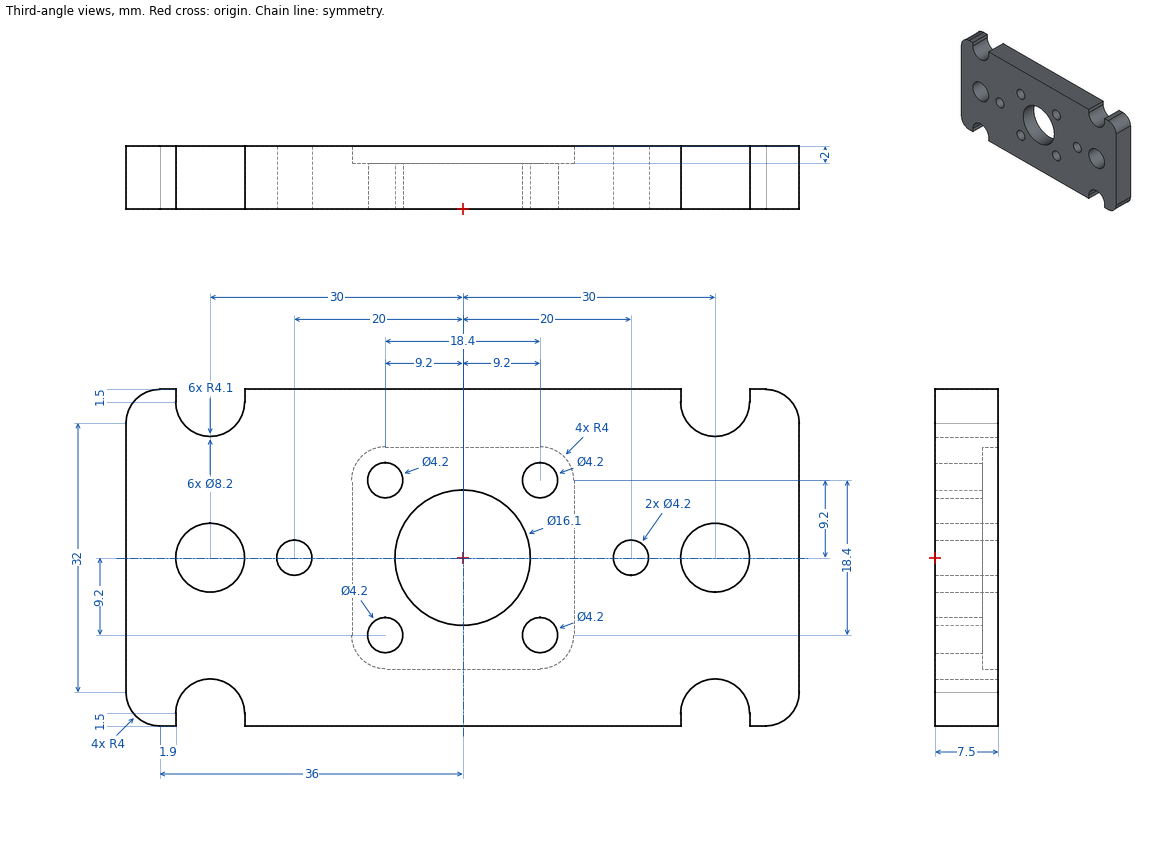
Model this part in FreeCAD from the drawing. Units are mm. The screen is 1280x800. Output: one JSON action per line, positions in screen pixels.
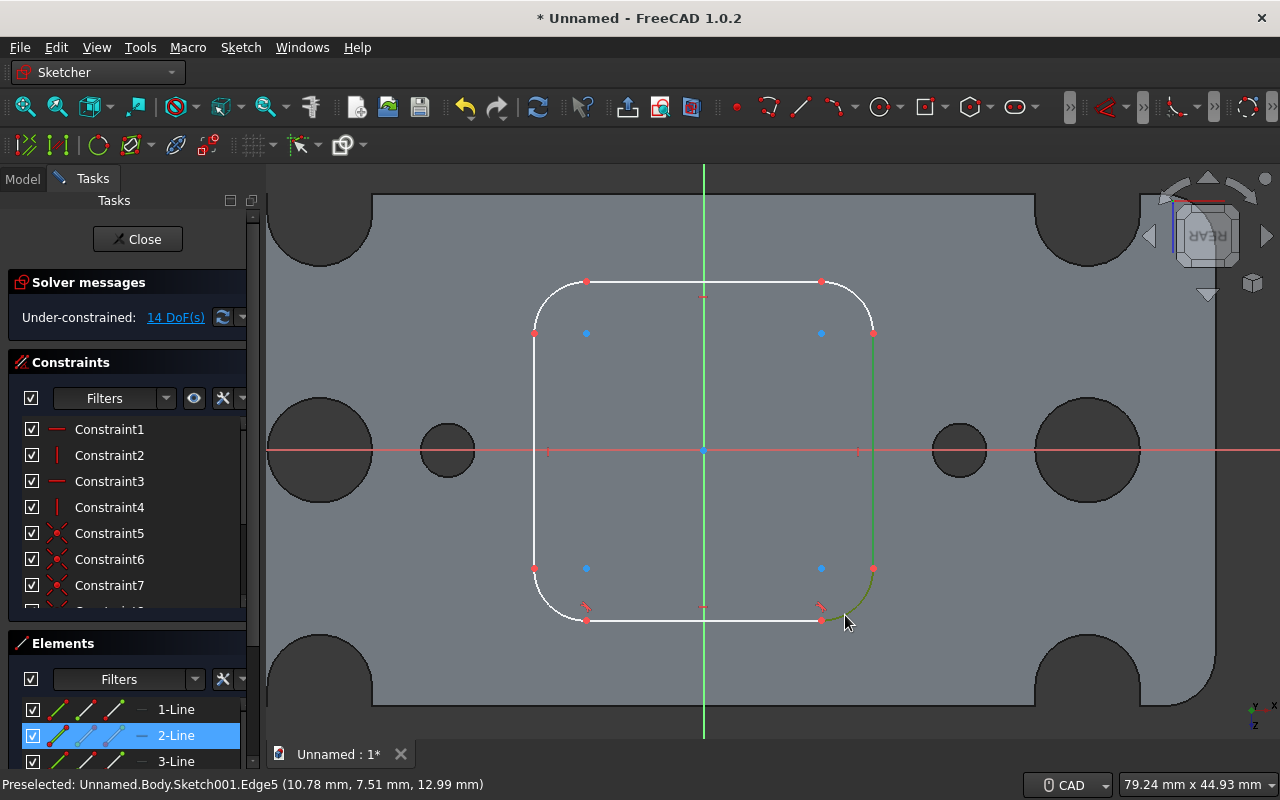
{"action": "key", "text": "t"}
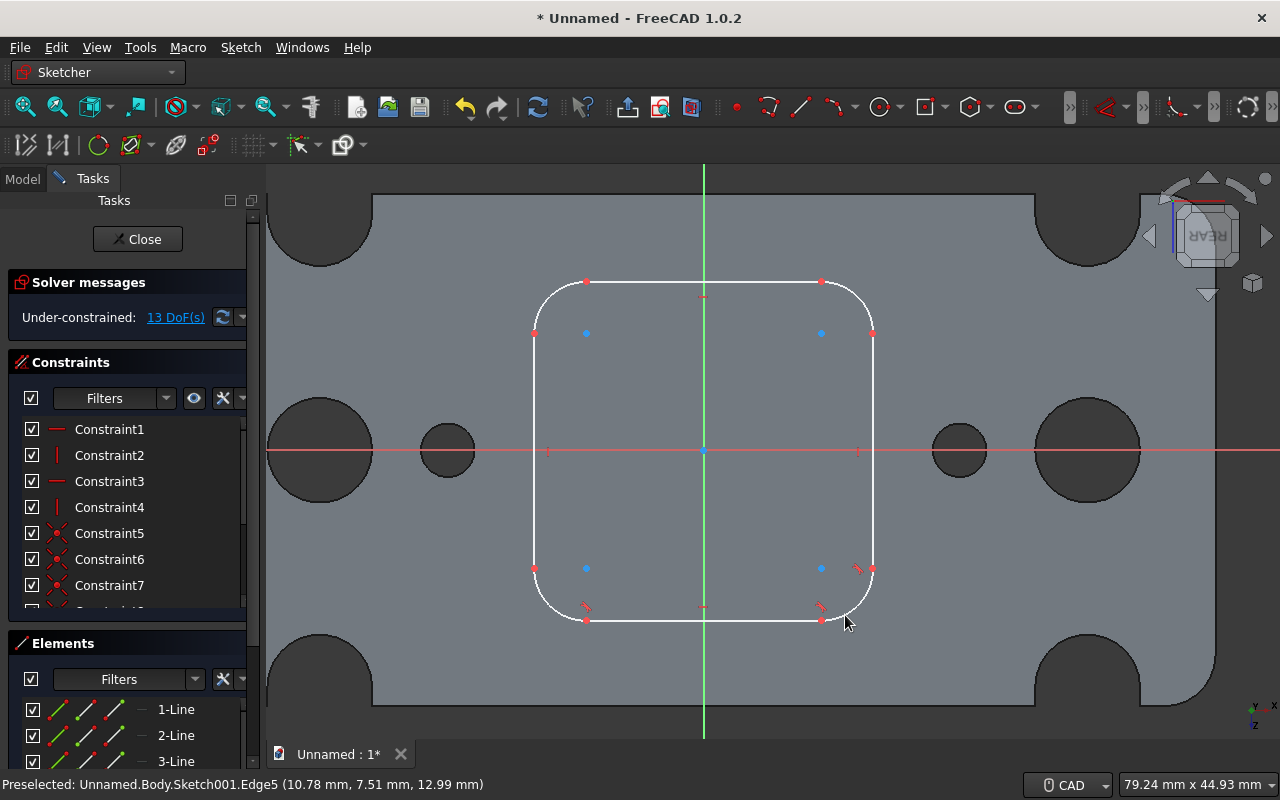
{"action": "left_click", "coordinate": [873, 498]}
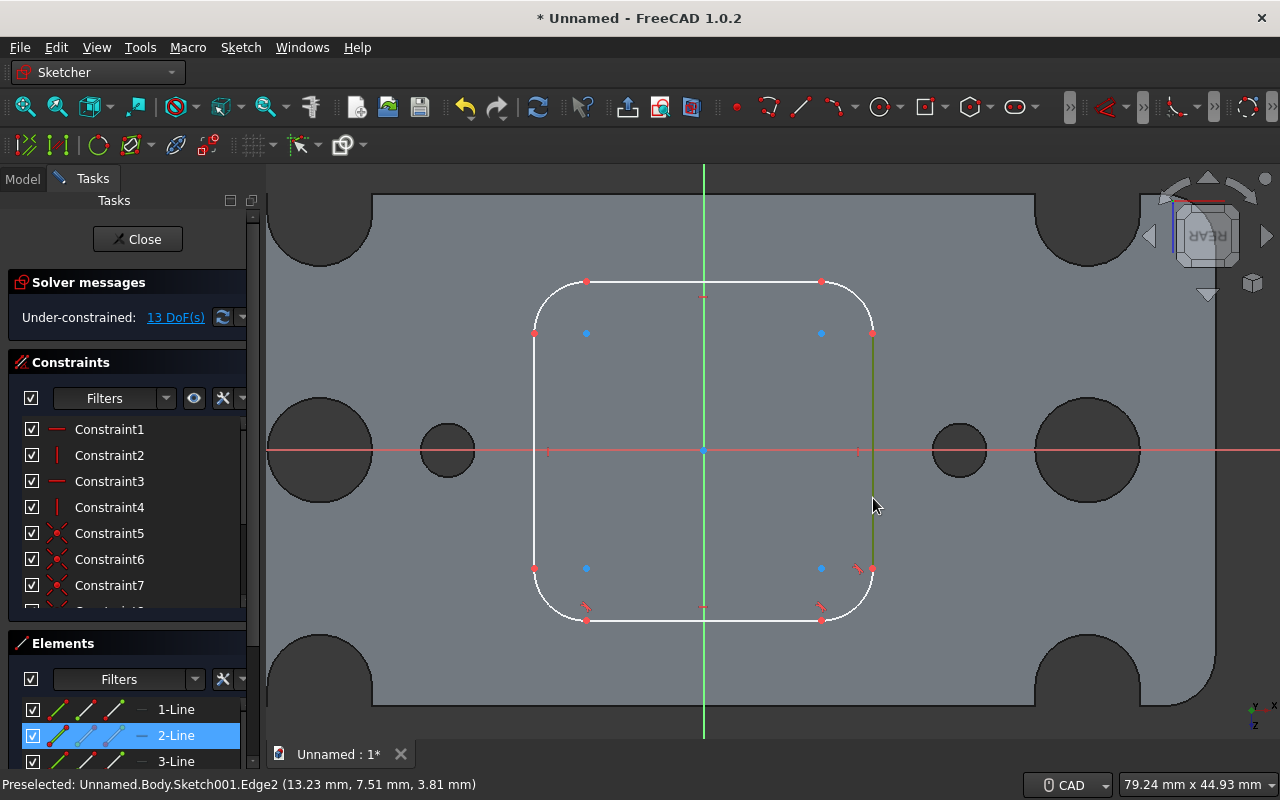
{"action": "left_click", "coordinate": [868, 310]}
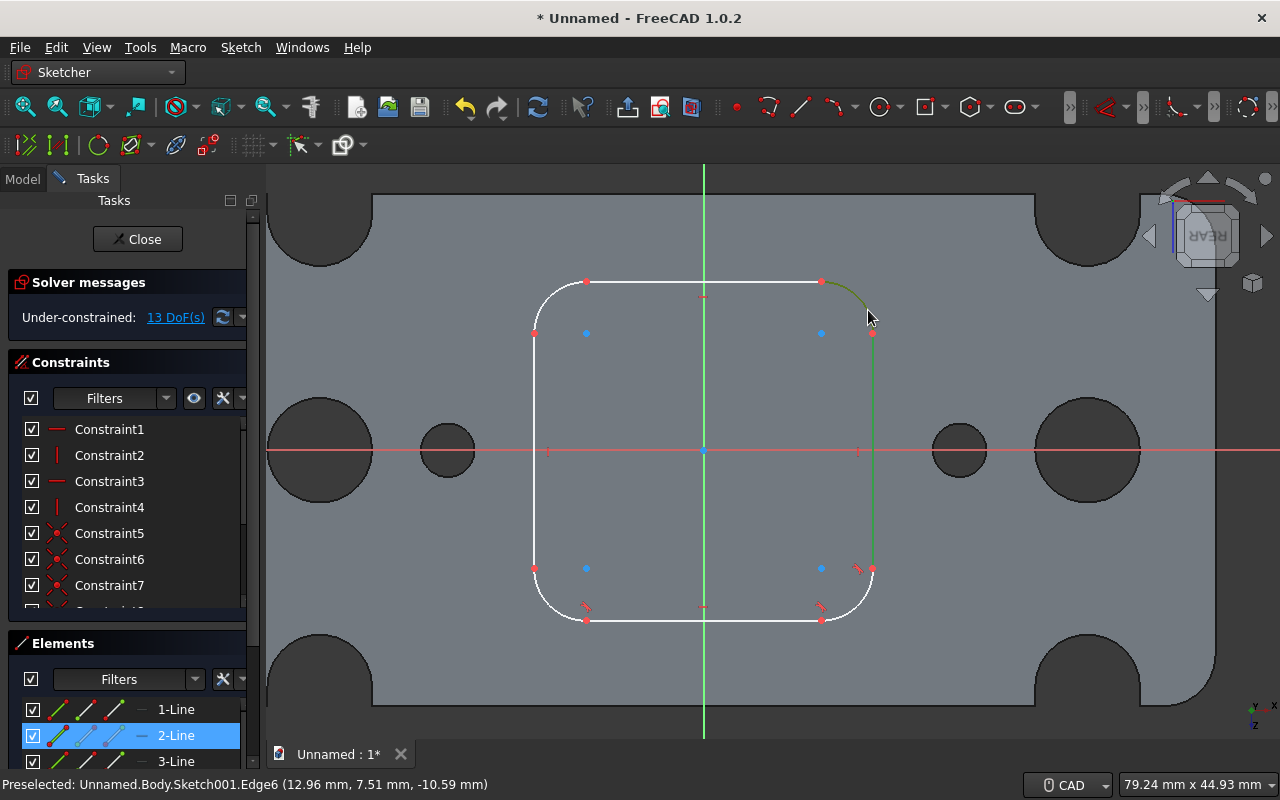
{"action": "key", "text": "t"}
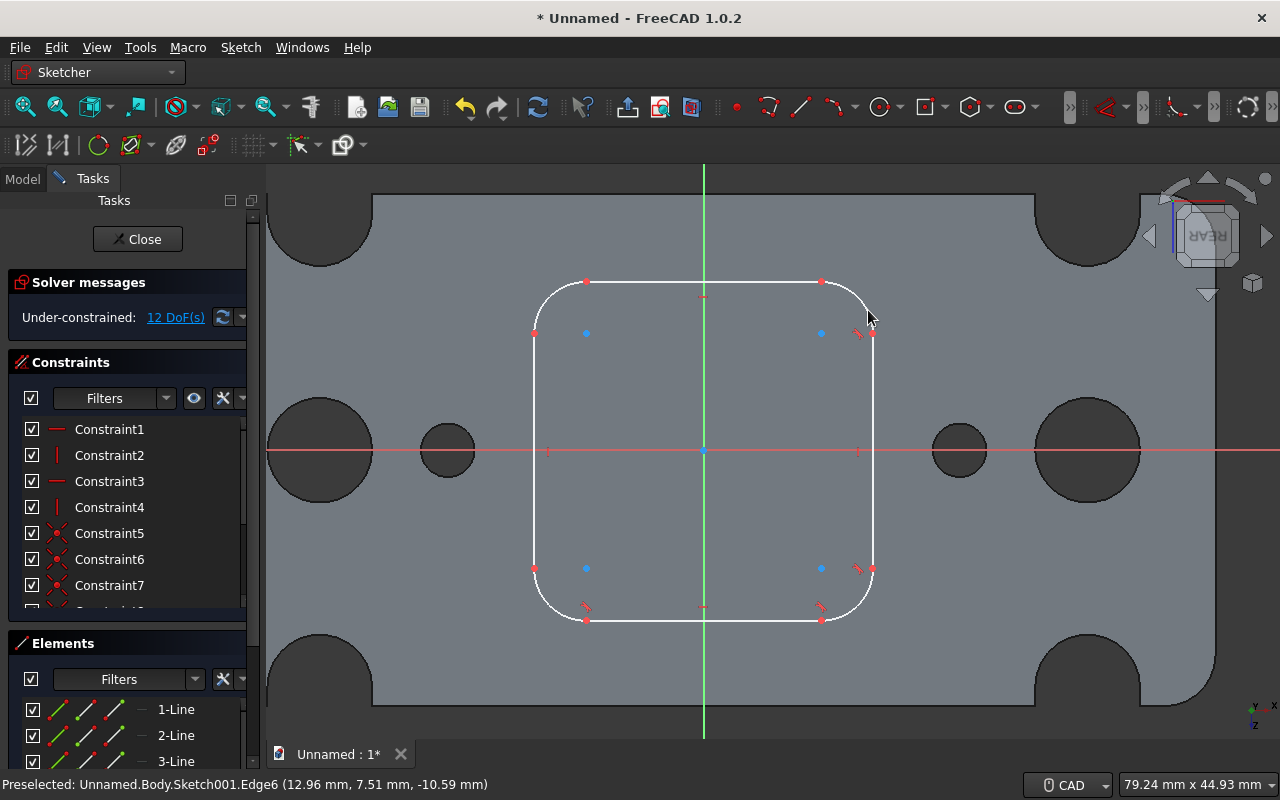
{"action": "left_click", "coordinate": [750, 282]}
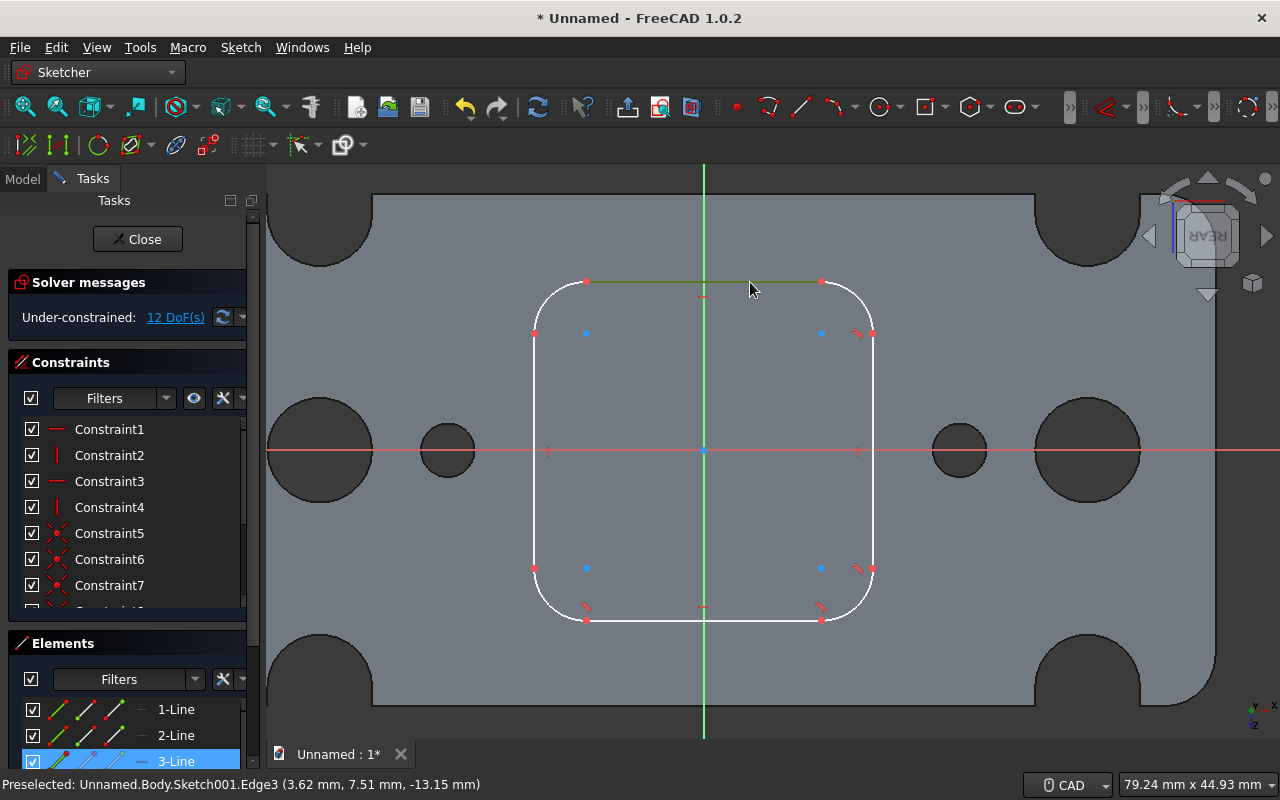
{"action": "left_click", "coordinate": [867, 310]}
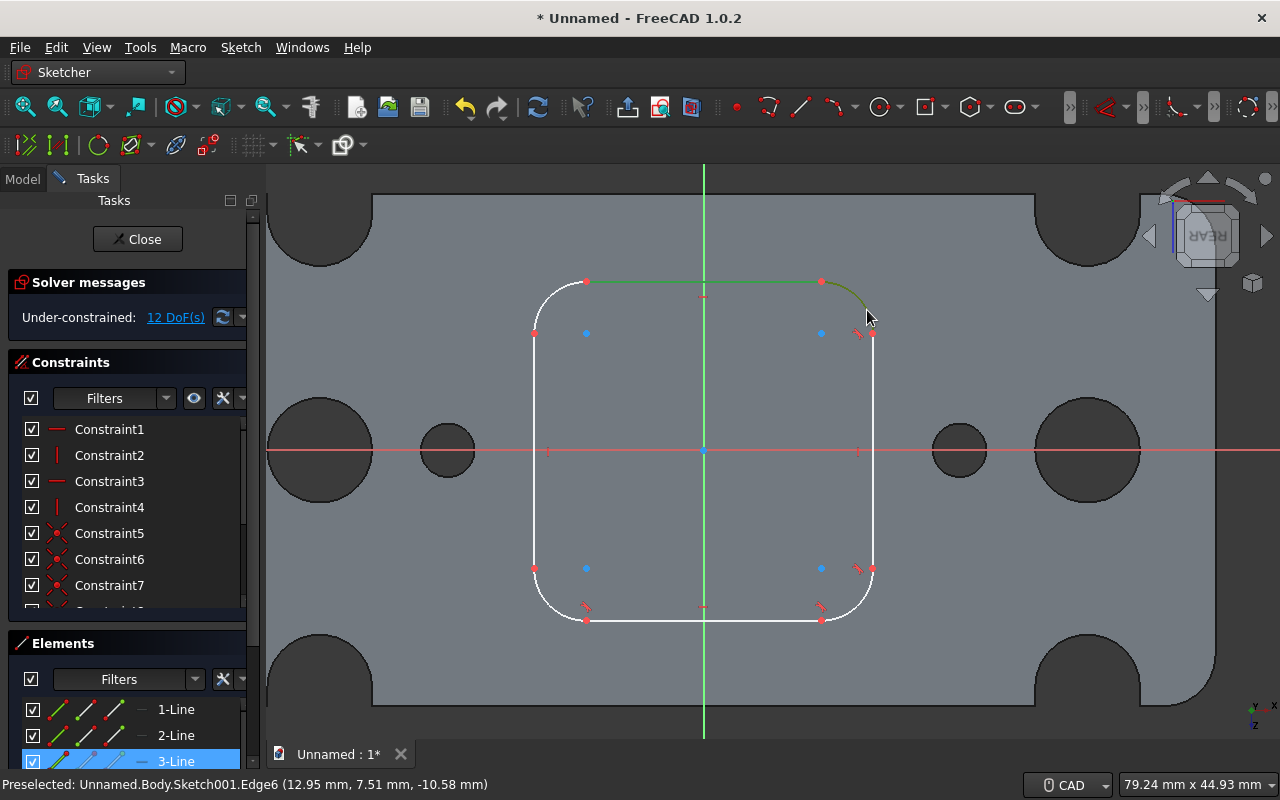
{"action": "key", "text": "t"}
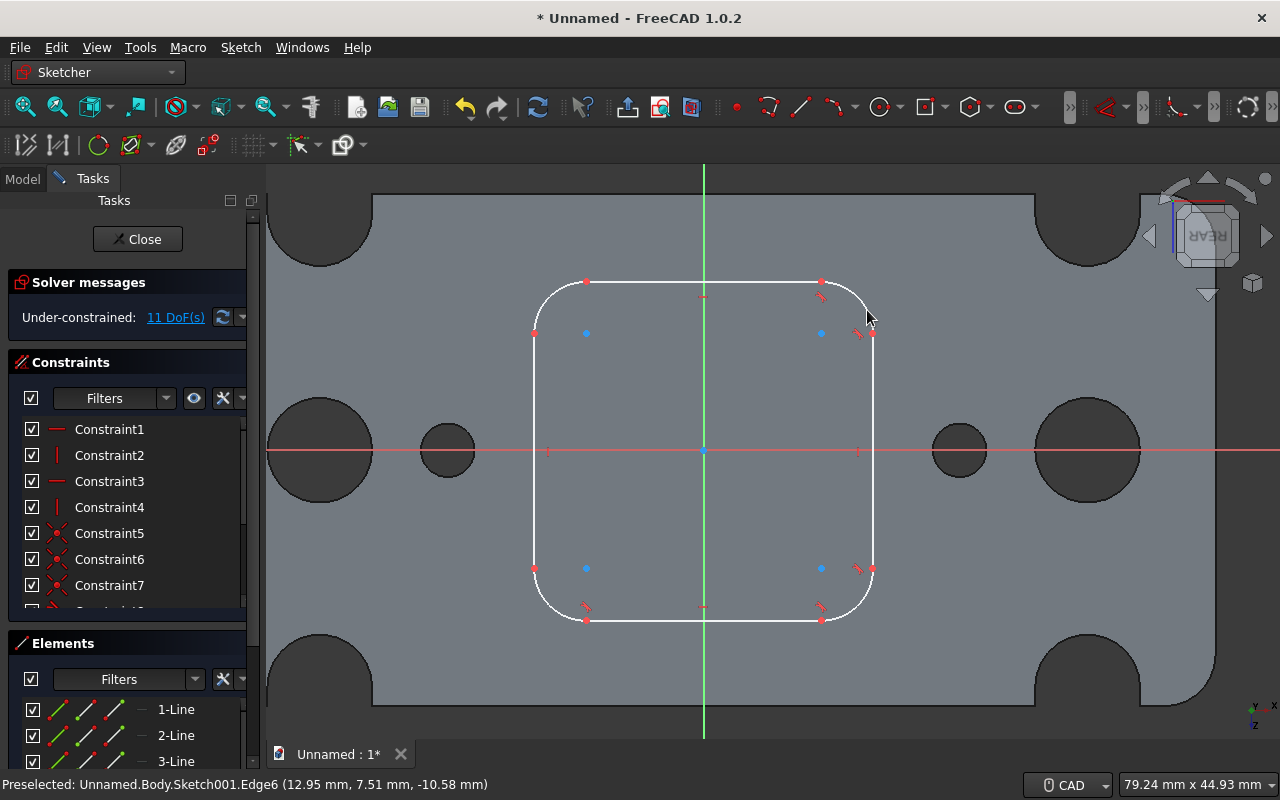
{"action": "left_click", "coordinate": [750, 282]}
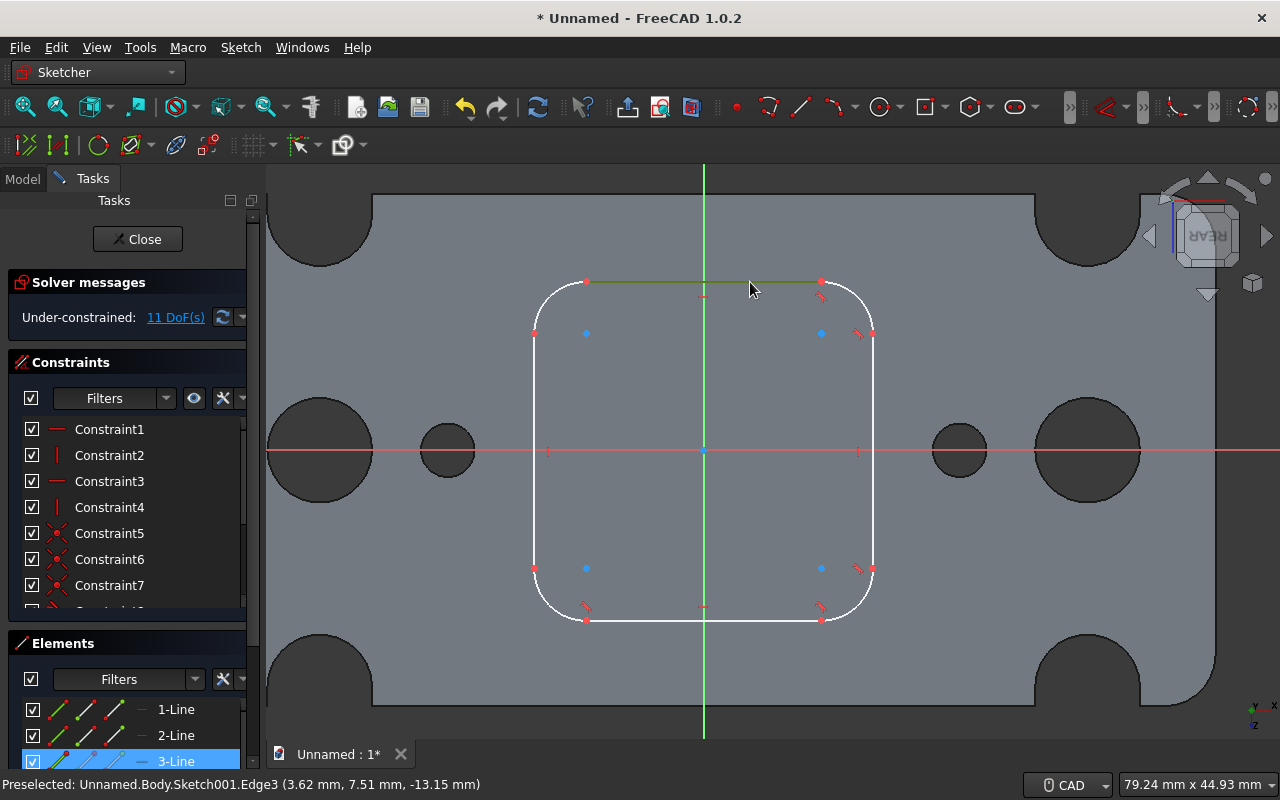
{"action": "left_click", "coordinate": [562, 288]}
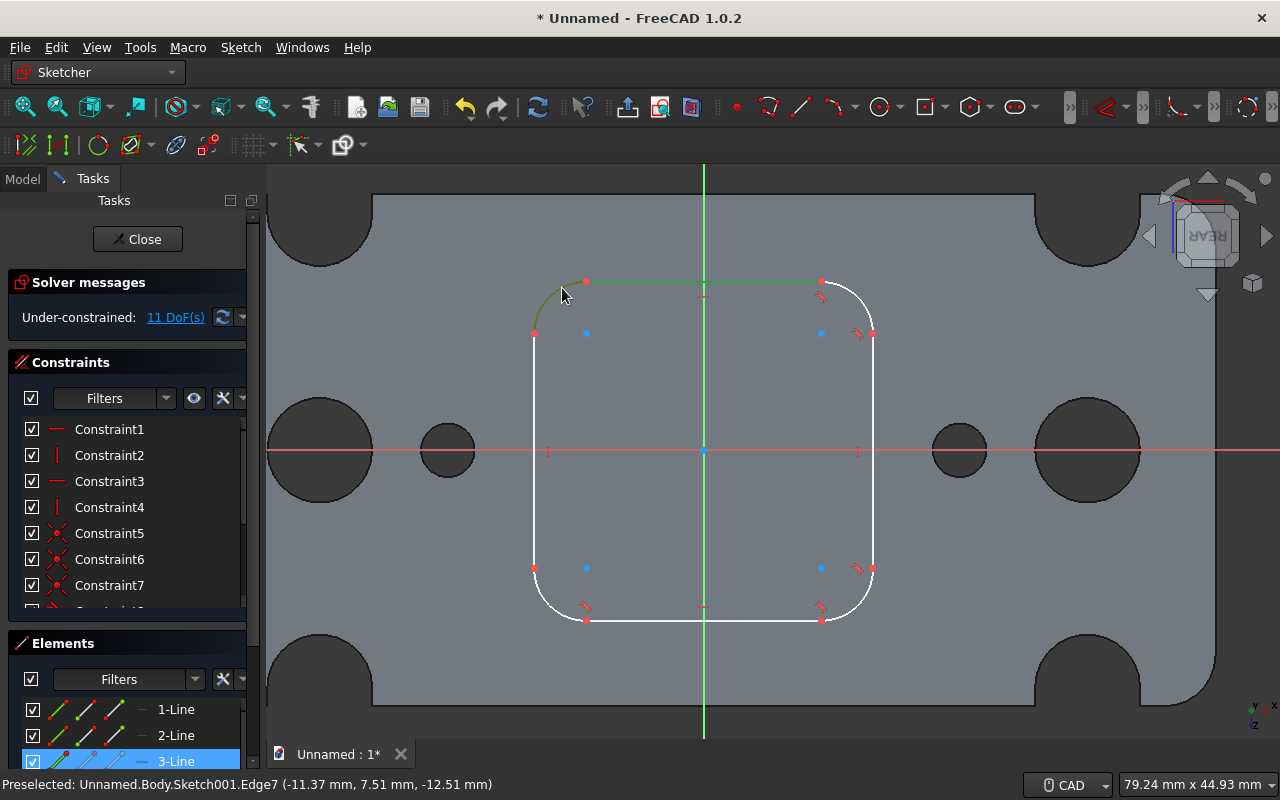
{"action": "key", "text": "t"}